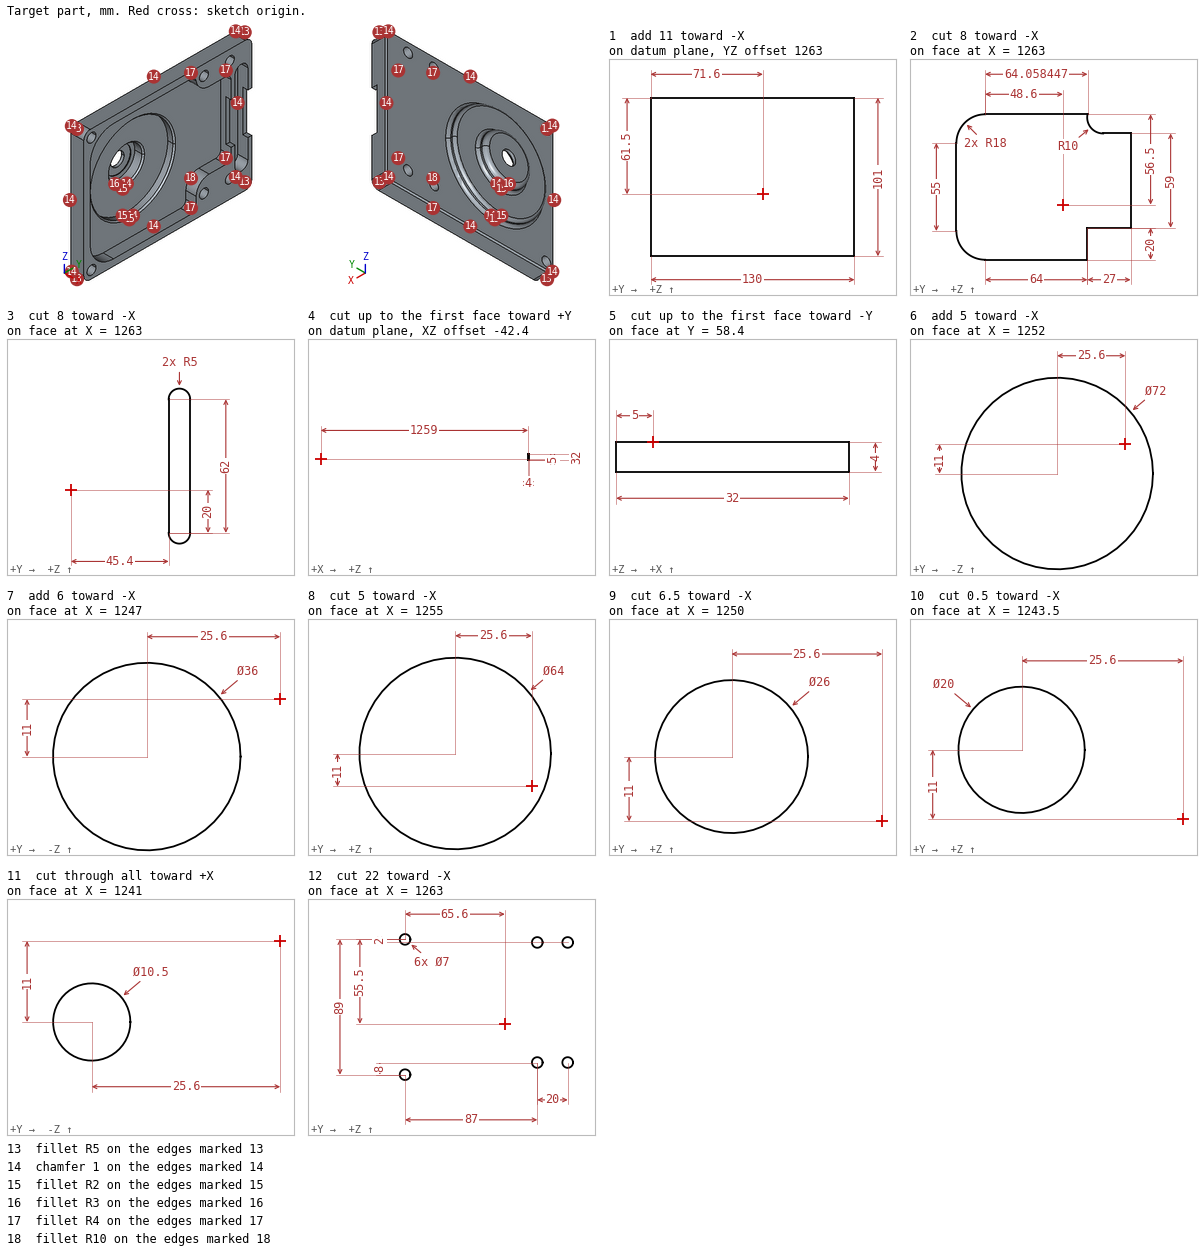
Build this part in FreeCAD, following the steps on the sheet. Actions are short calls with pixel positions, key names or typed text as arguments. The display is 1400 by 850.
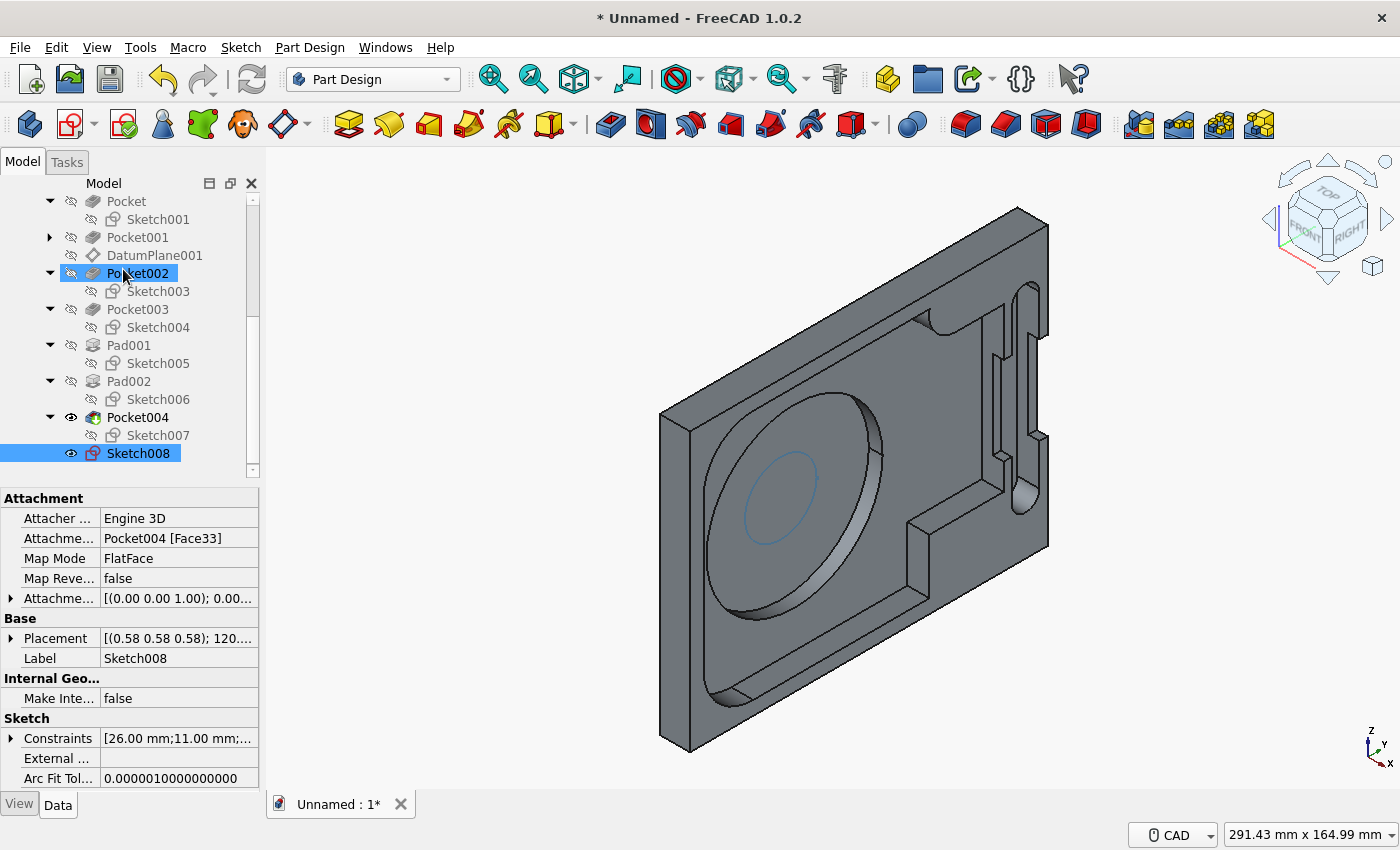
click(612, 124)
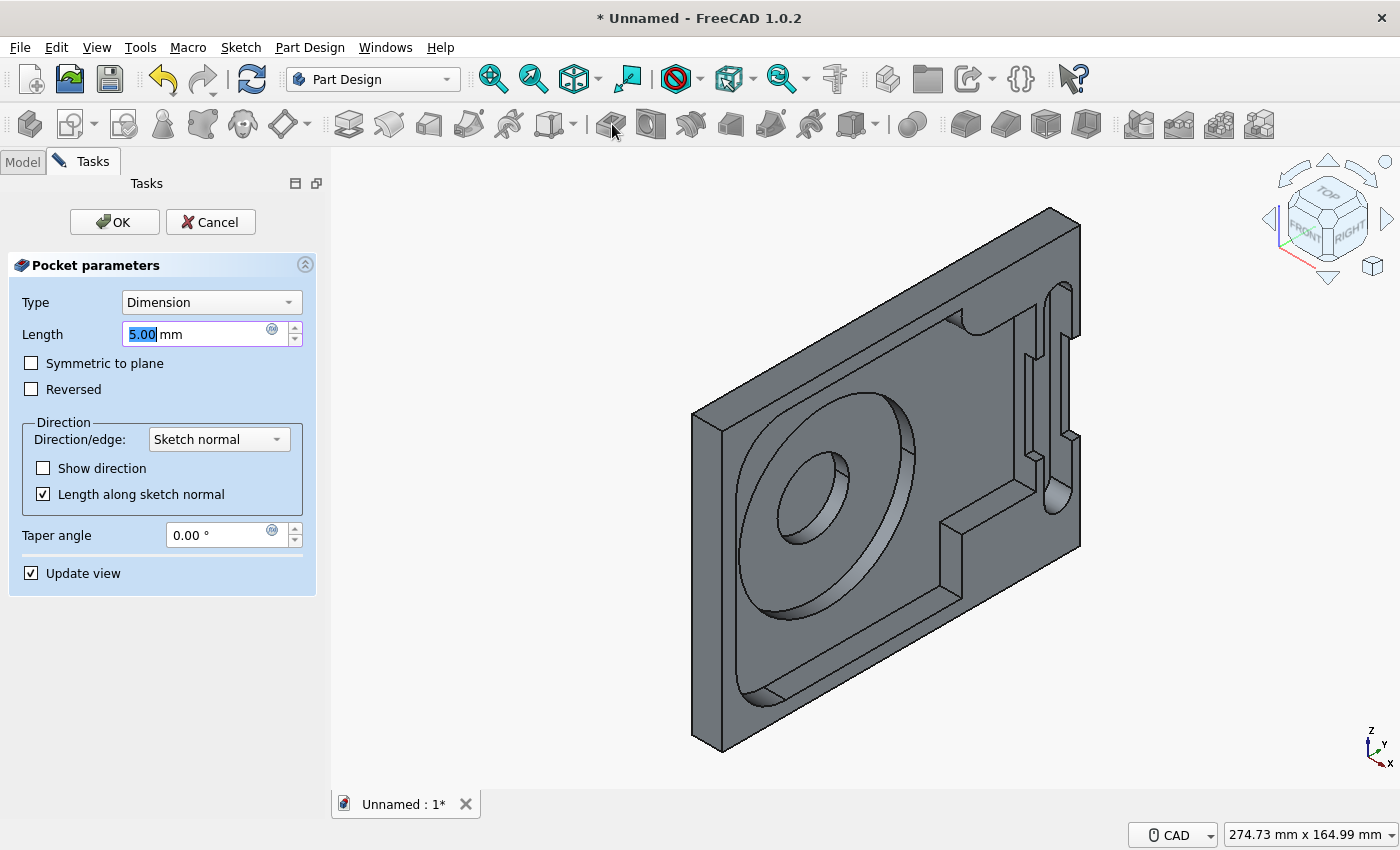
text(6.5)
key(Tab)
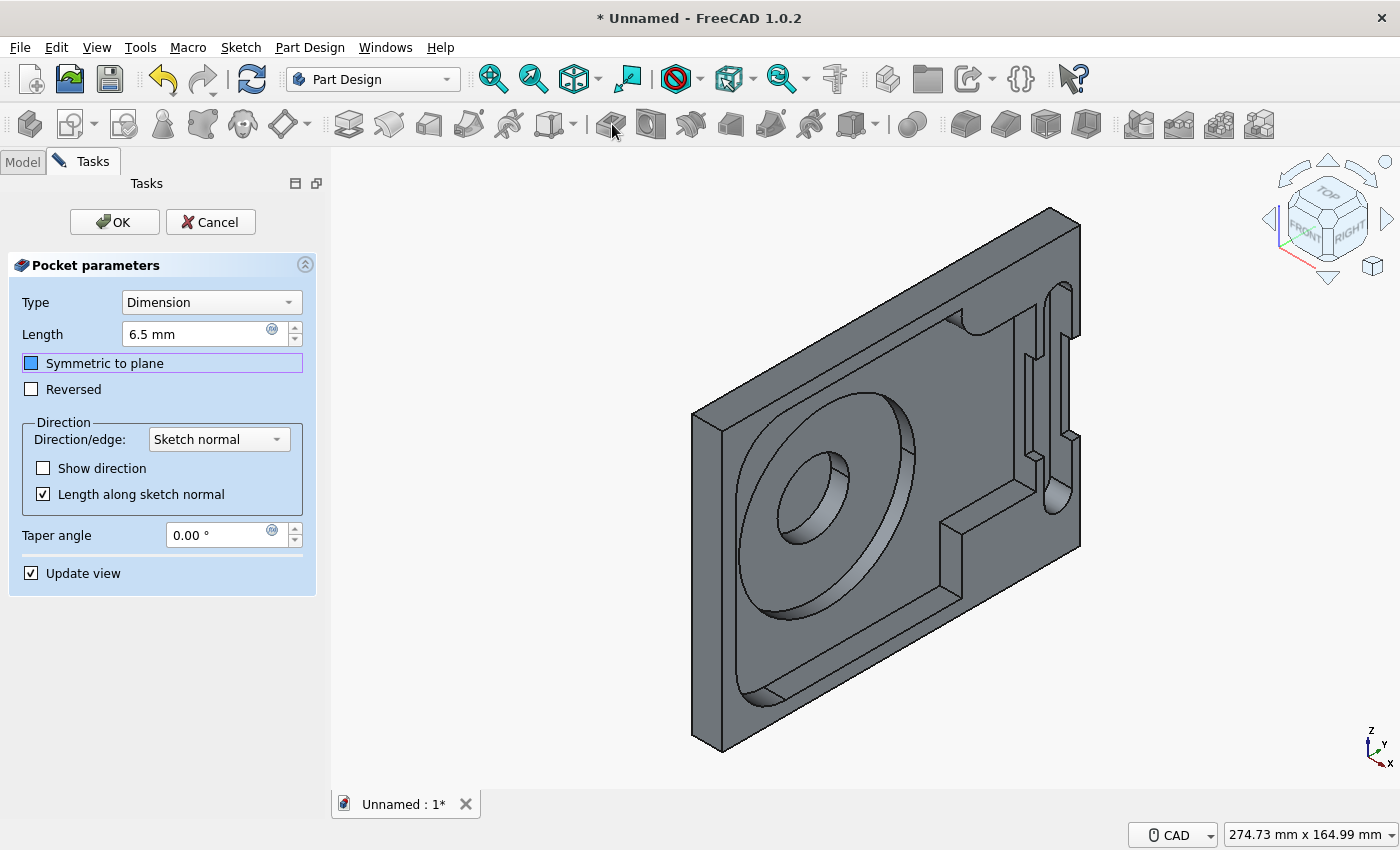
click(115, 222)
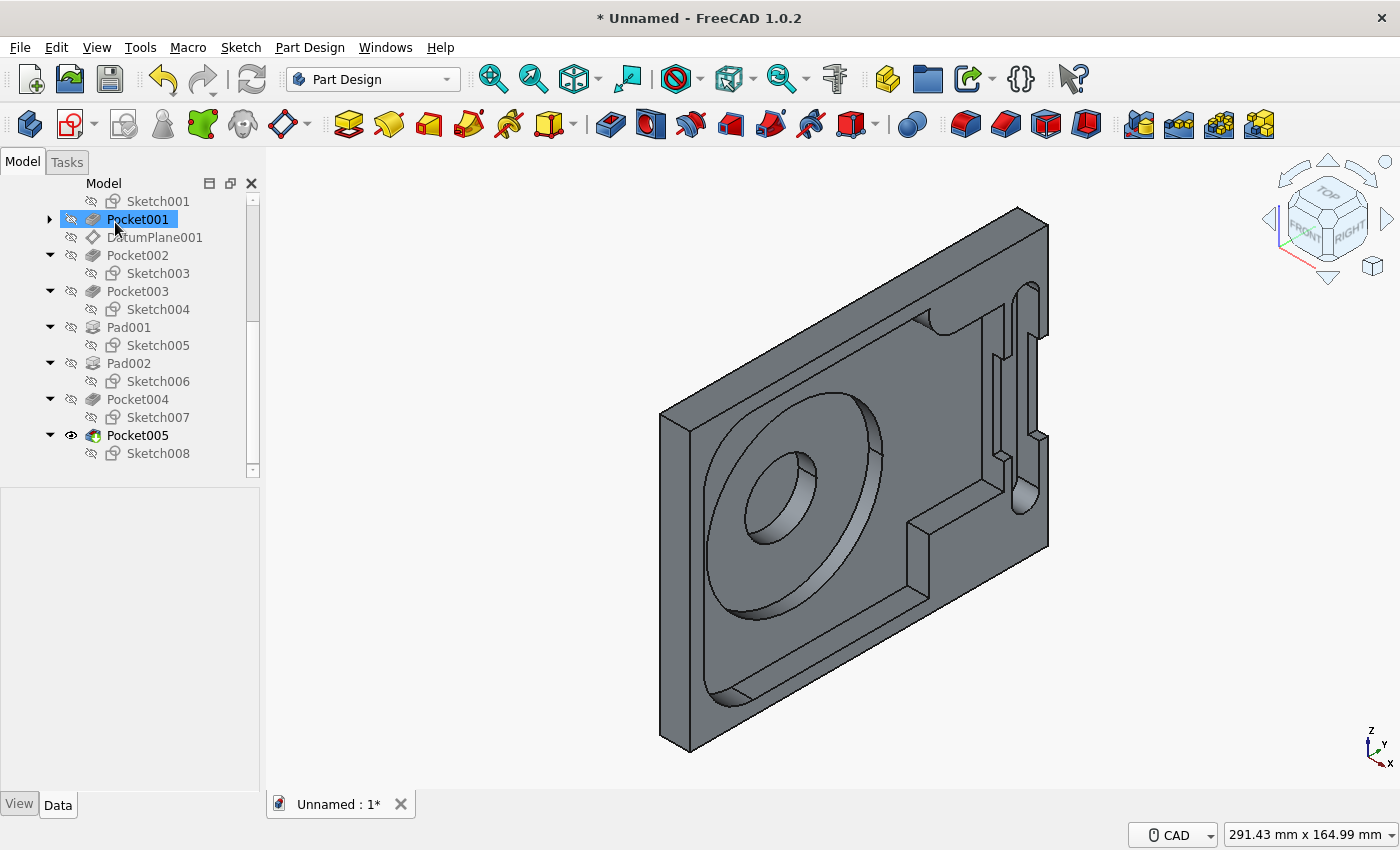
click(763, 499)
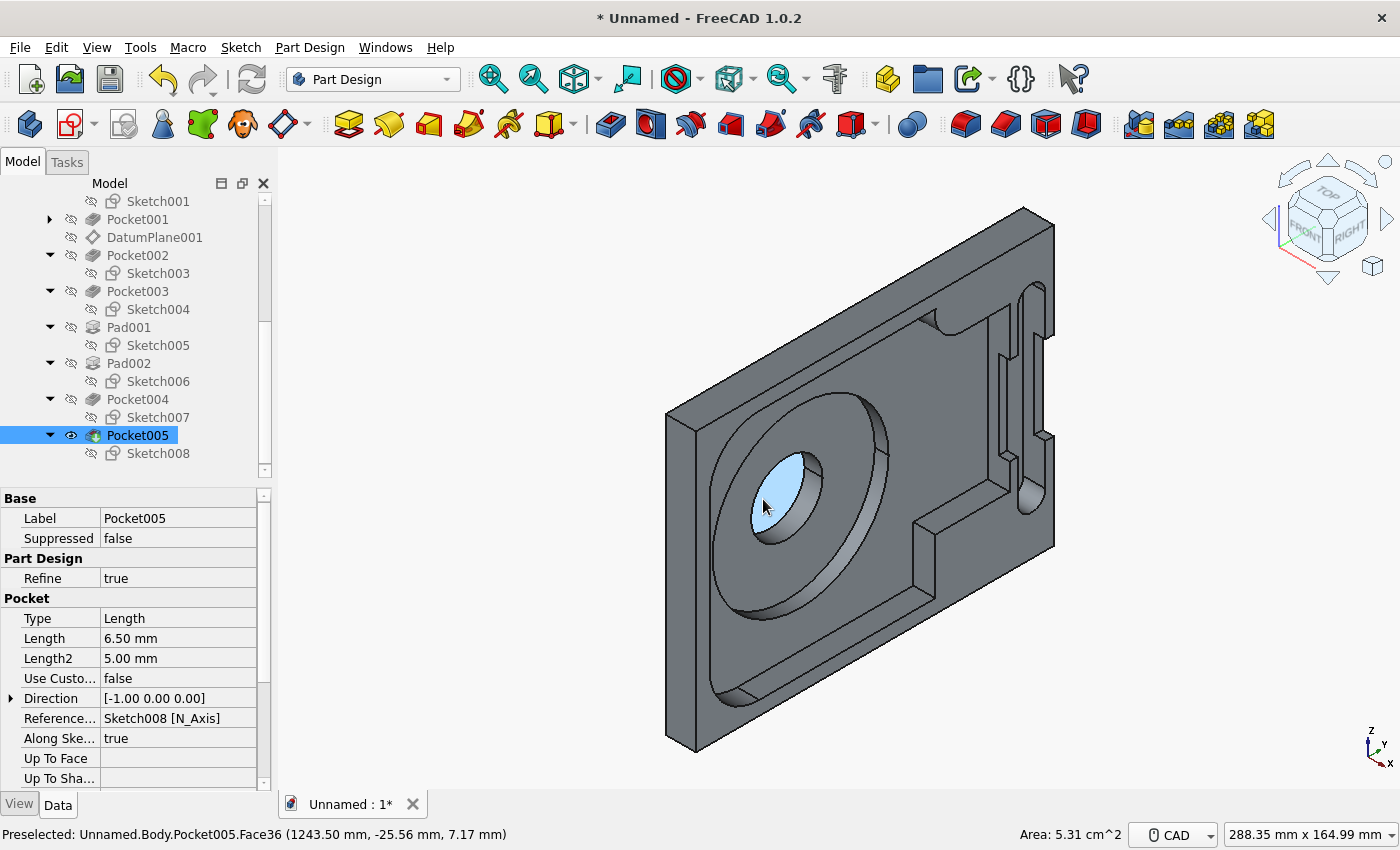
click(70, 124)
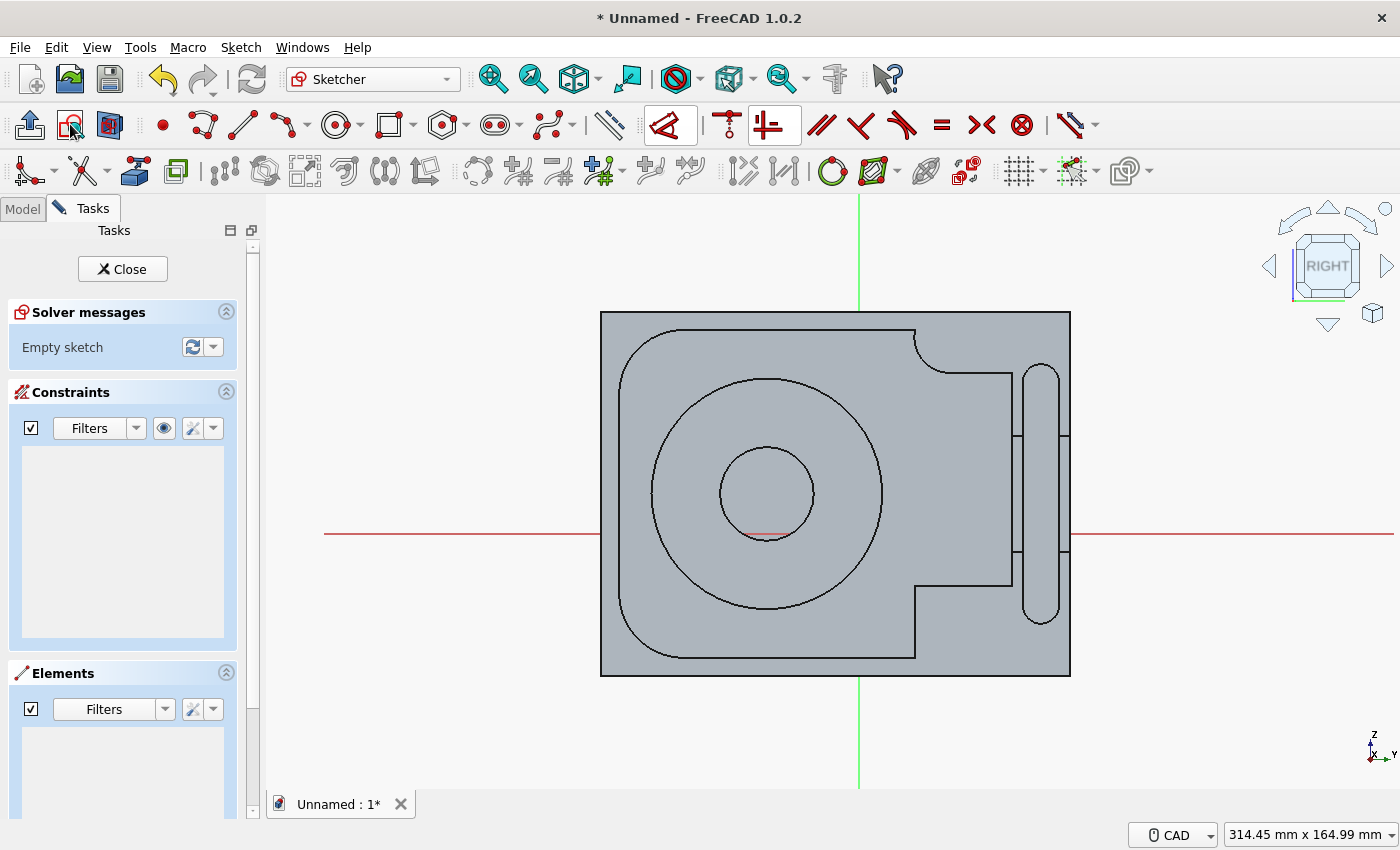
scroll(803, 497, up, 8)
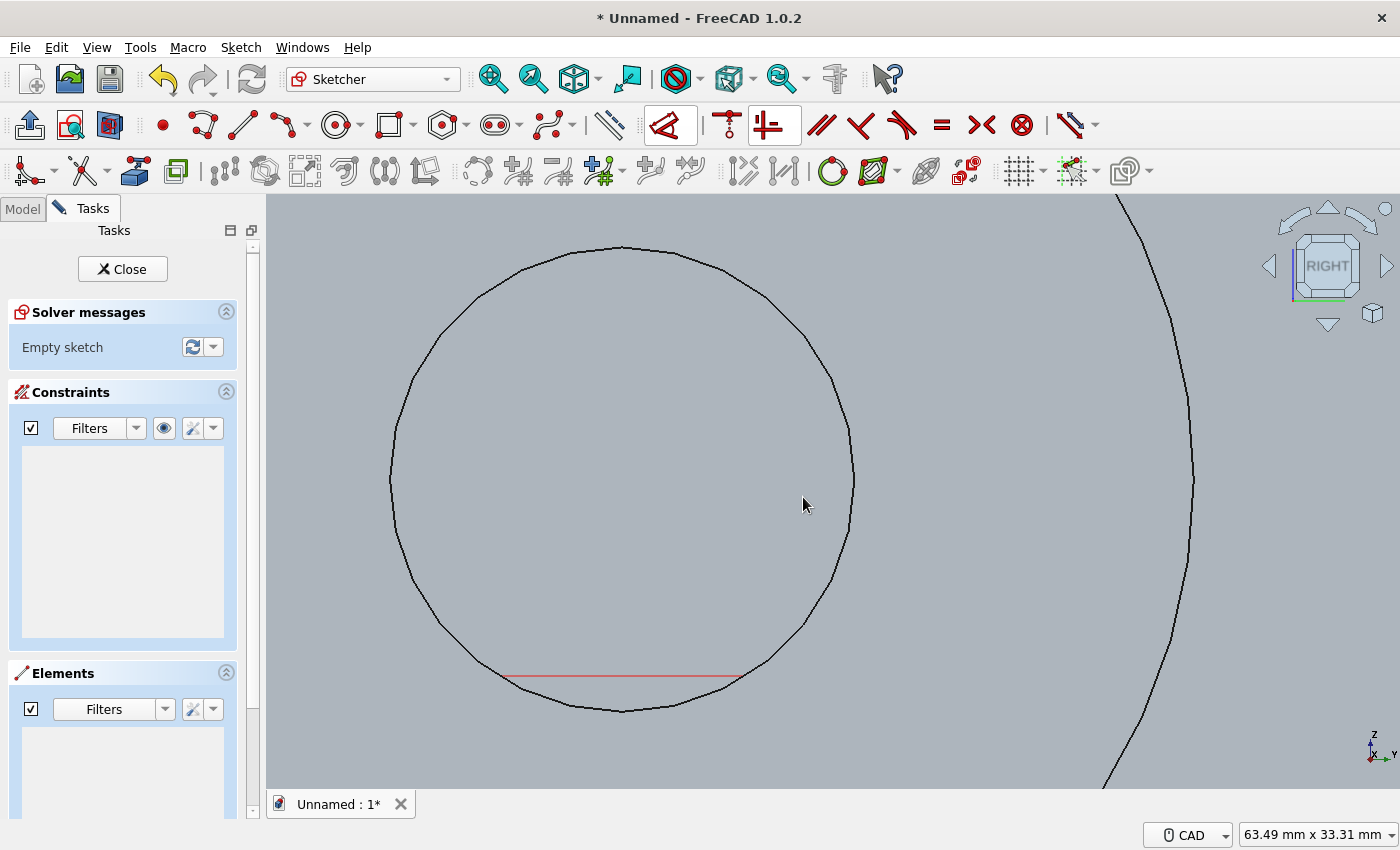
key(g)
key(c)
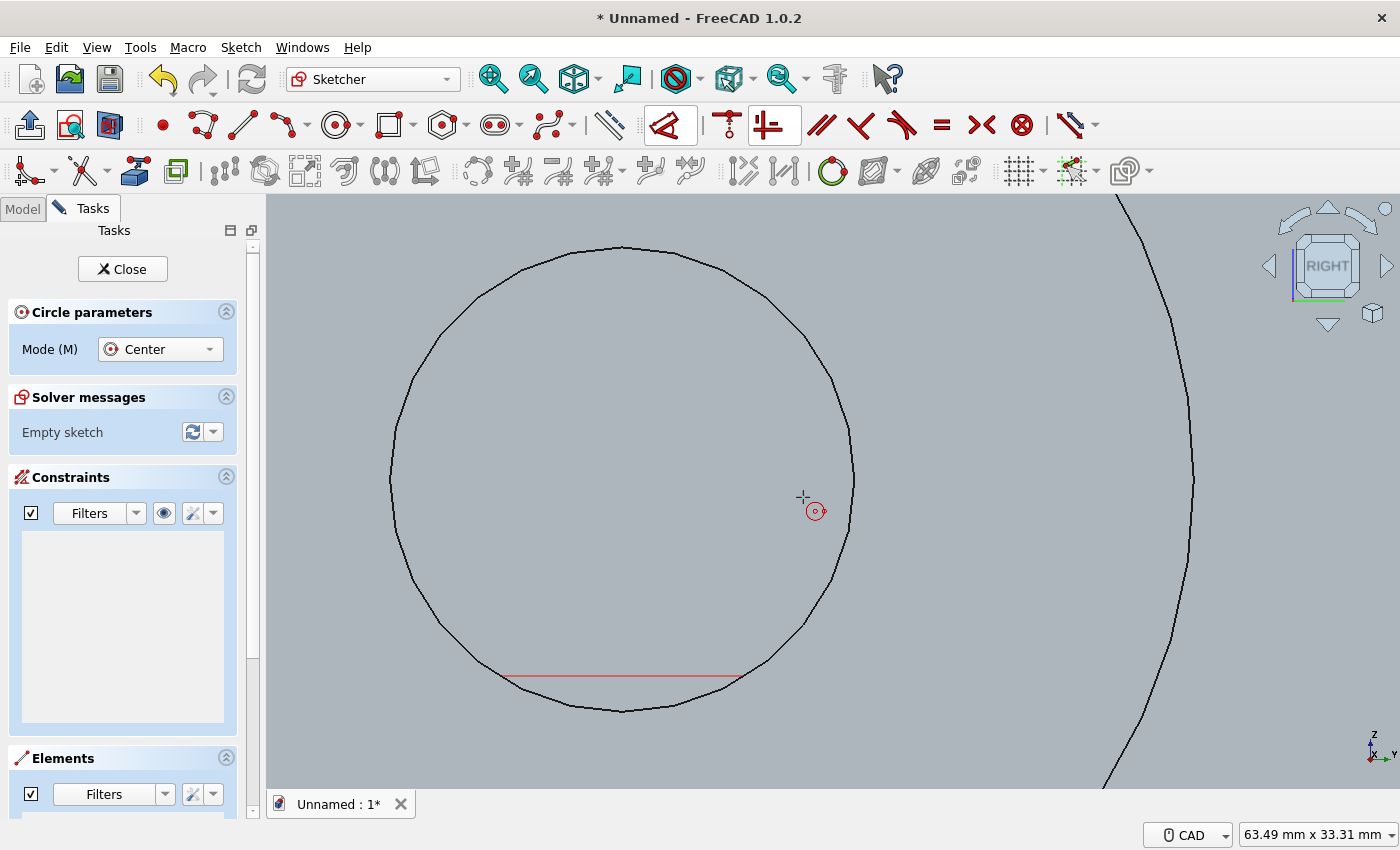
click(622, 480)
move(749, 353)